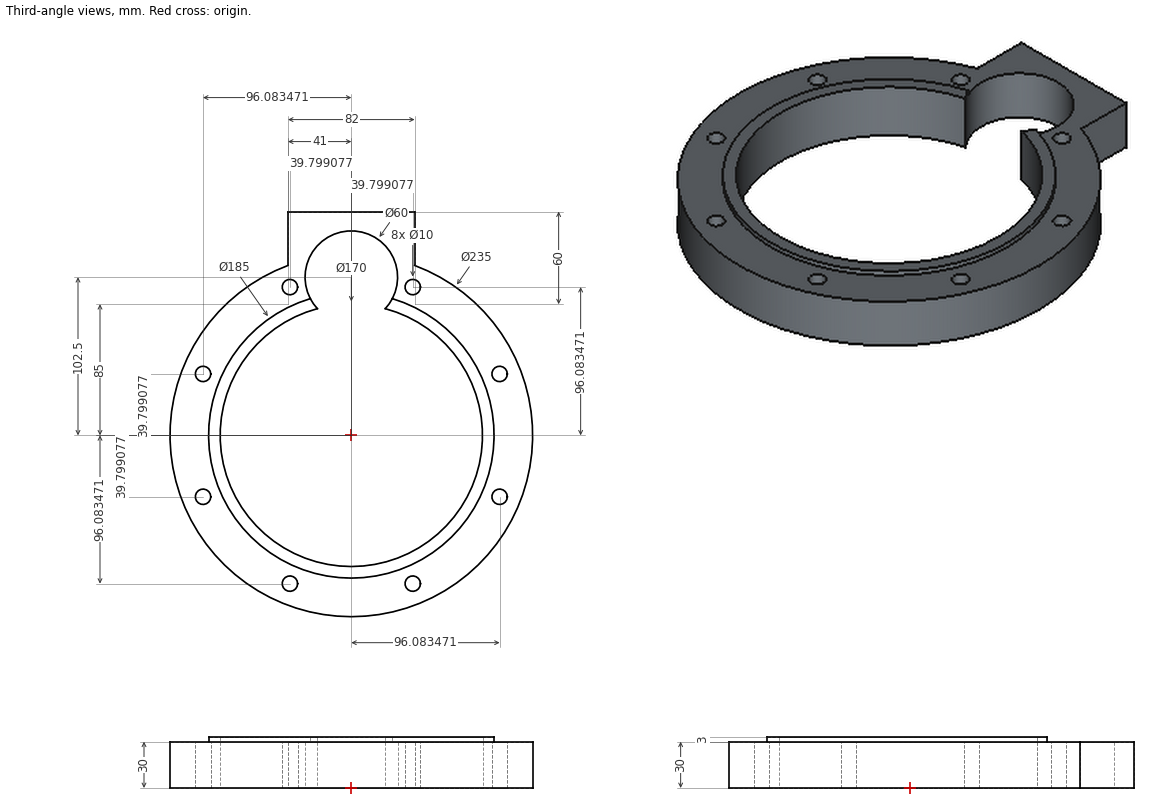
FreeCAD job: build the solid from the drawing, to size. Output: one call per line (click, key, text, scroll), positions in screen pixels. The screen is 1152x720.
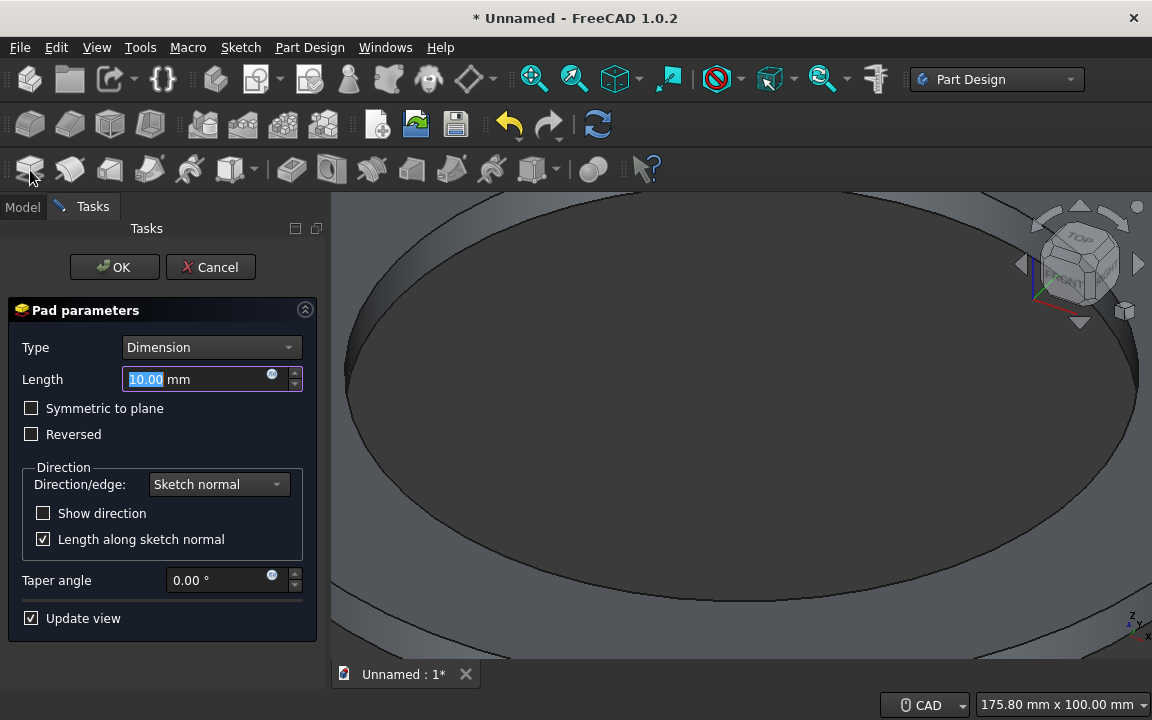
text(30)
key(Tab)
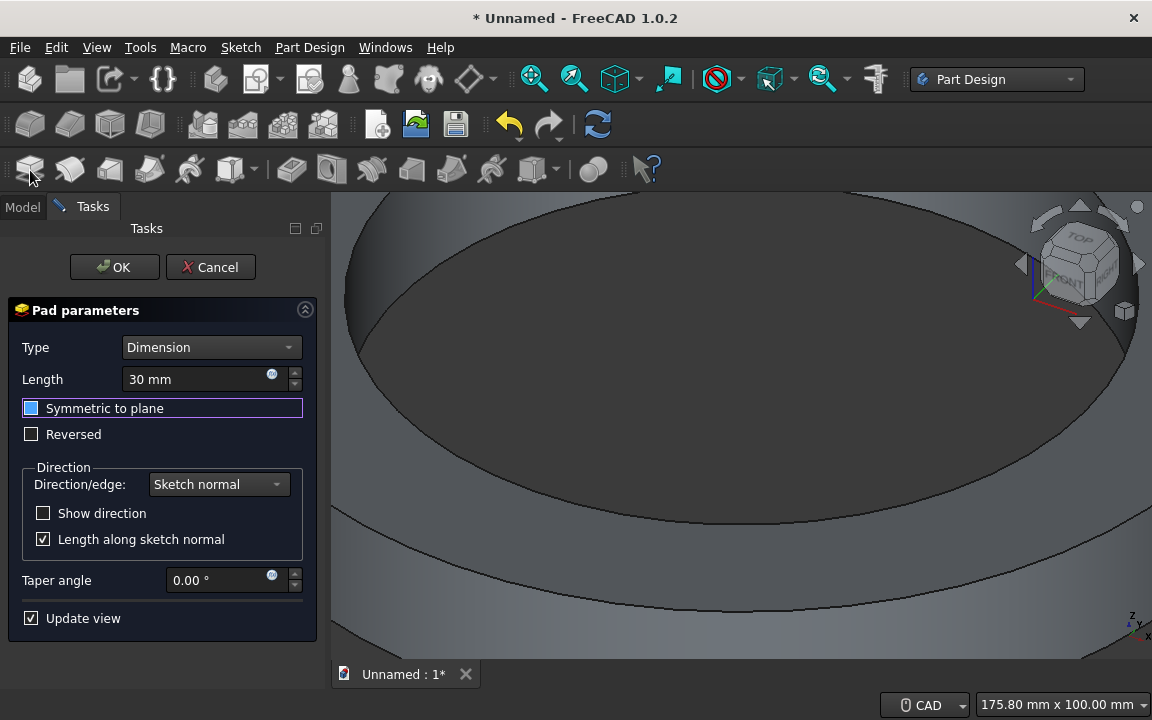
click(115, 267)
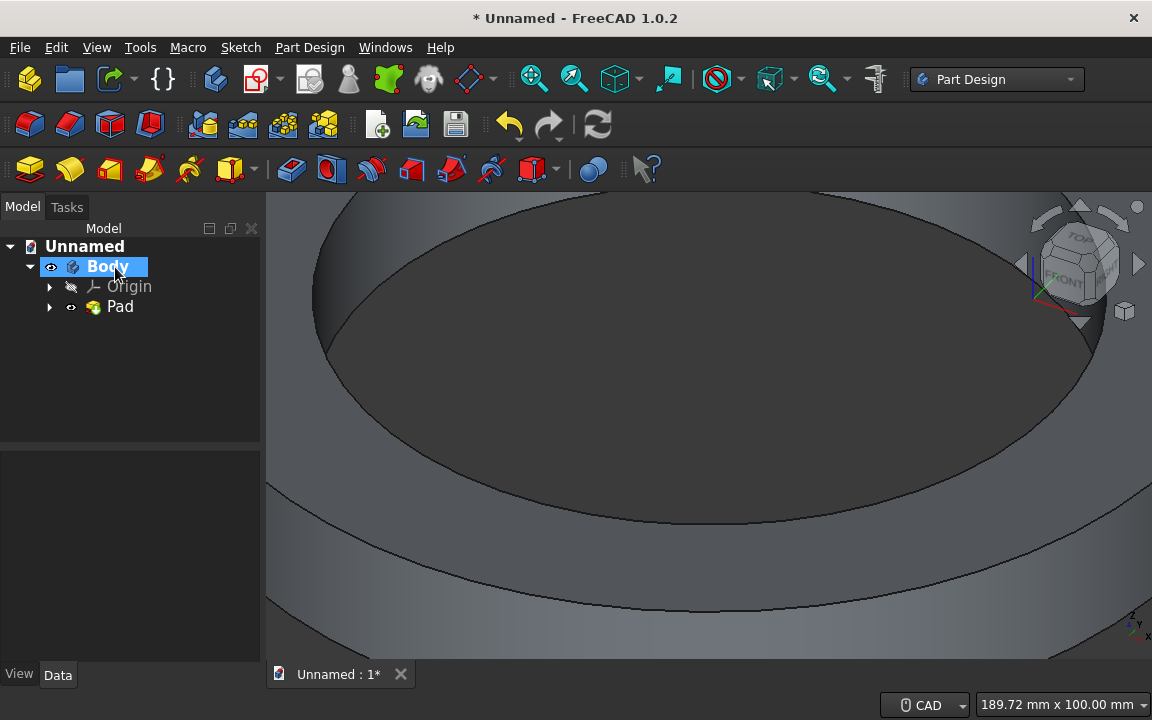
click(536, 80)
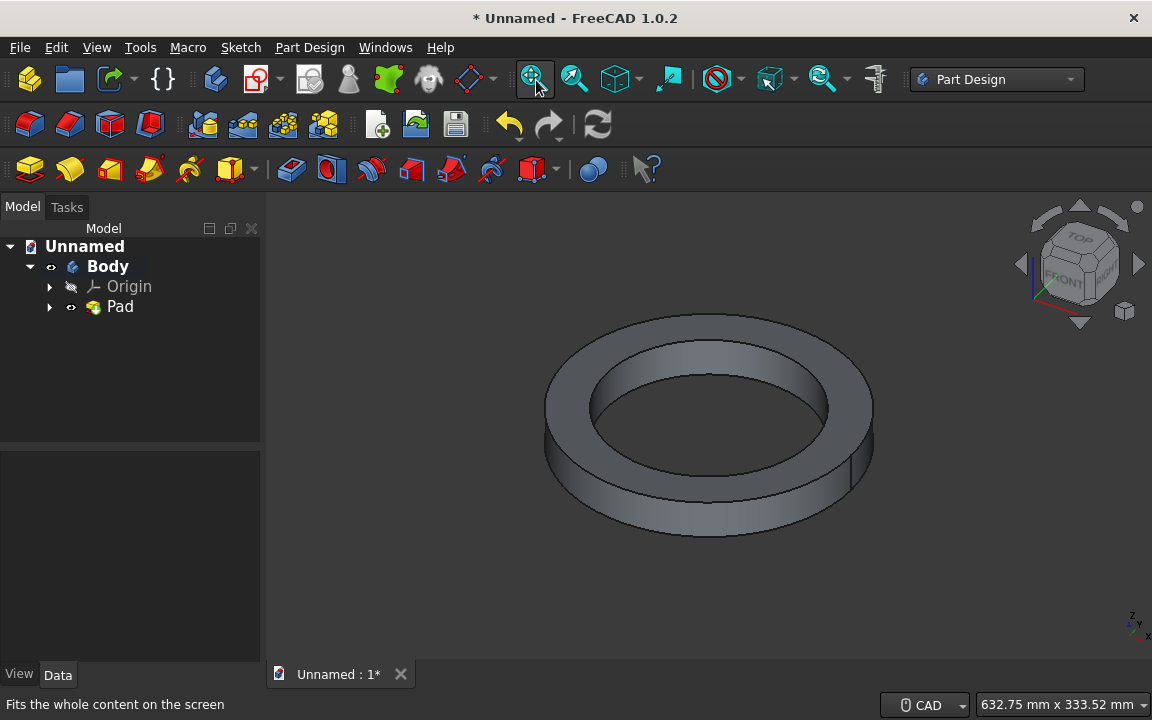
click(831, 448)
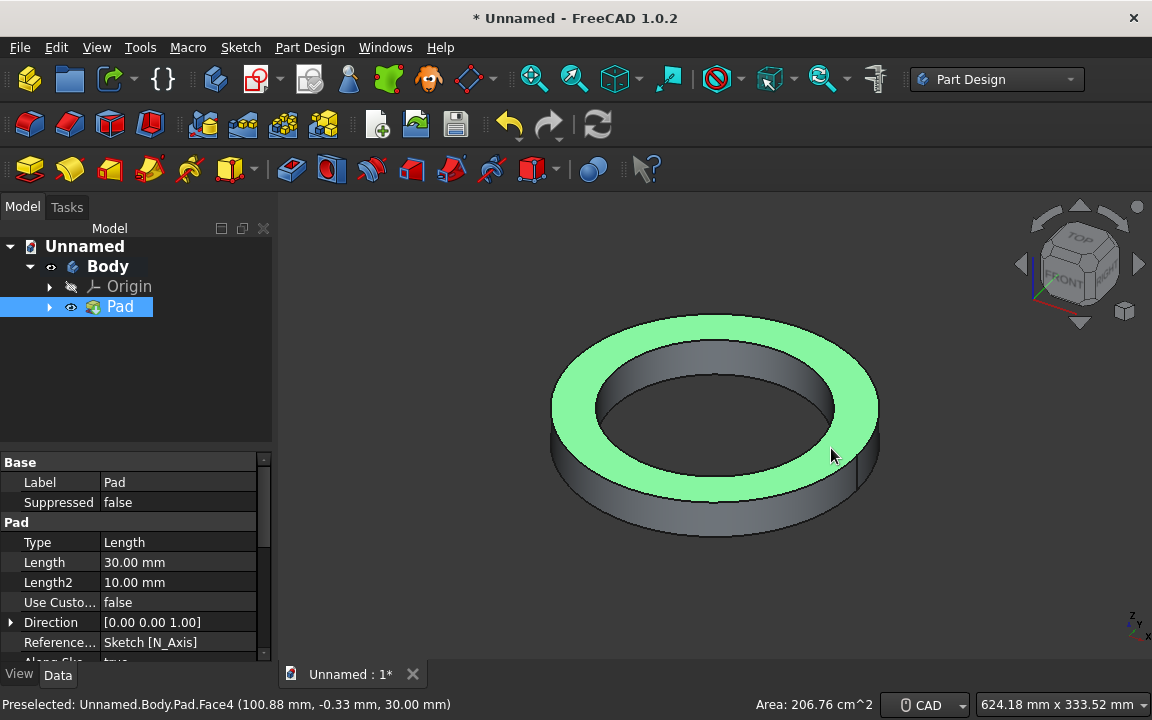
click(256, 80)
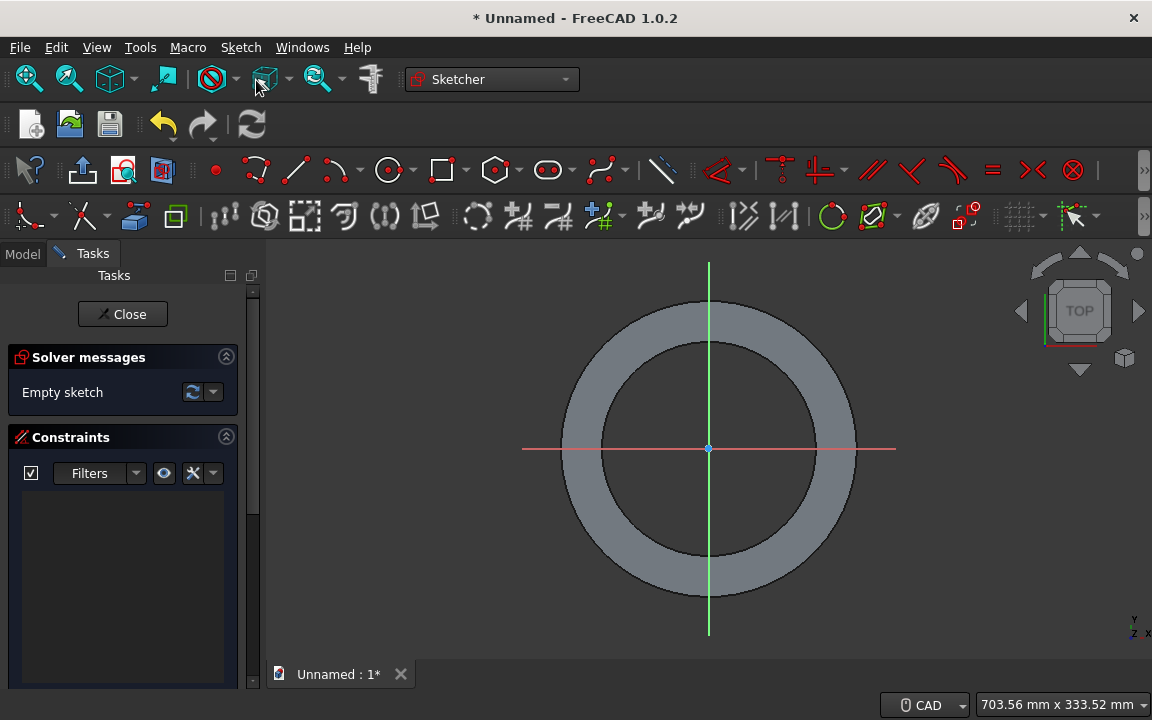
scroll(332, 631, down, 1)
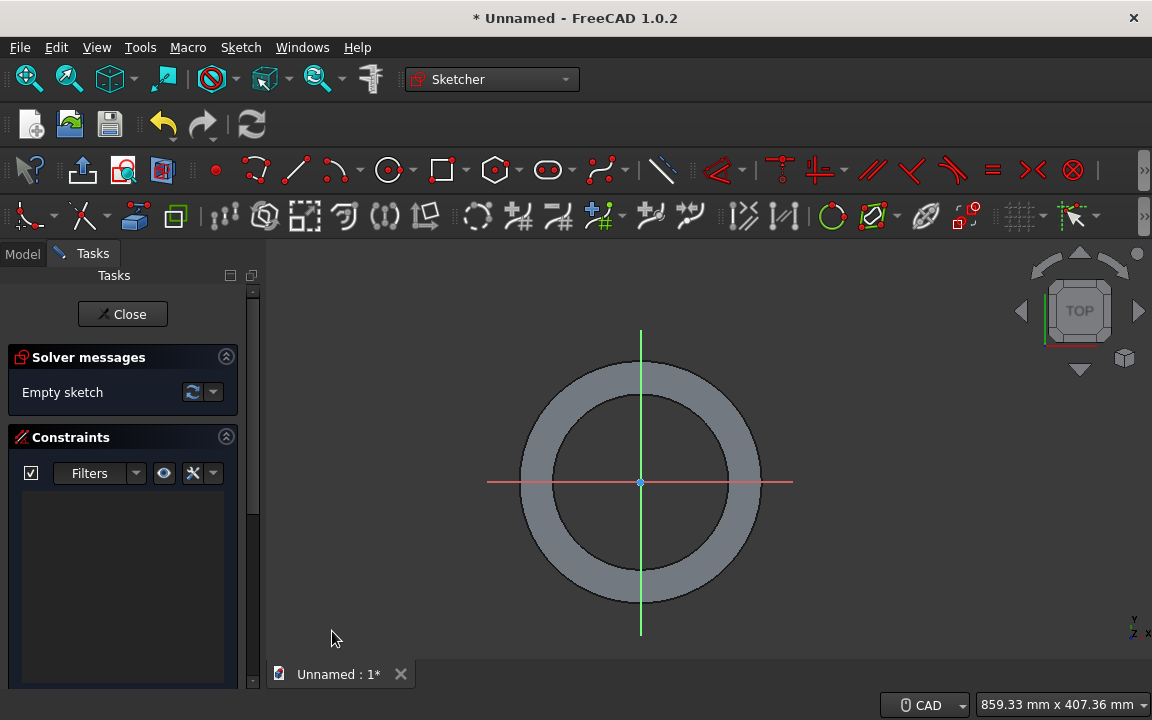
scroll(641, 357, up, 3)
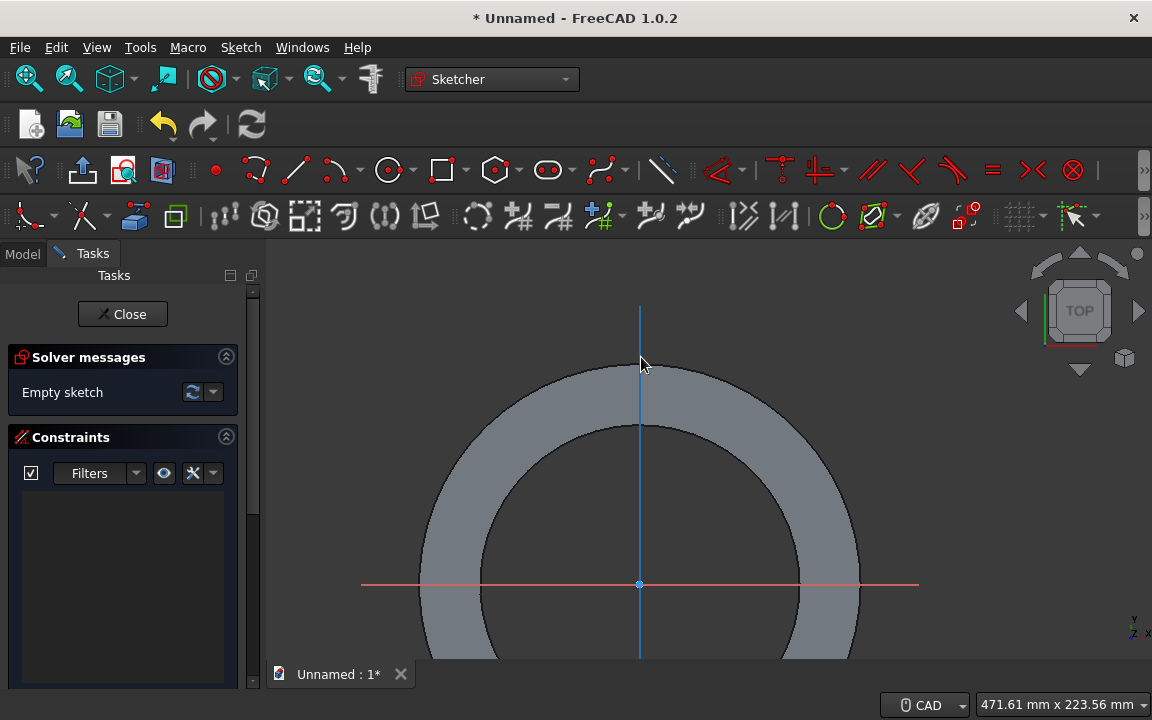
click(442, 170)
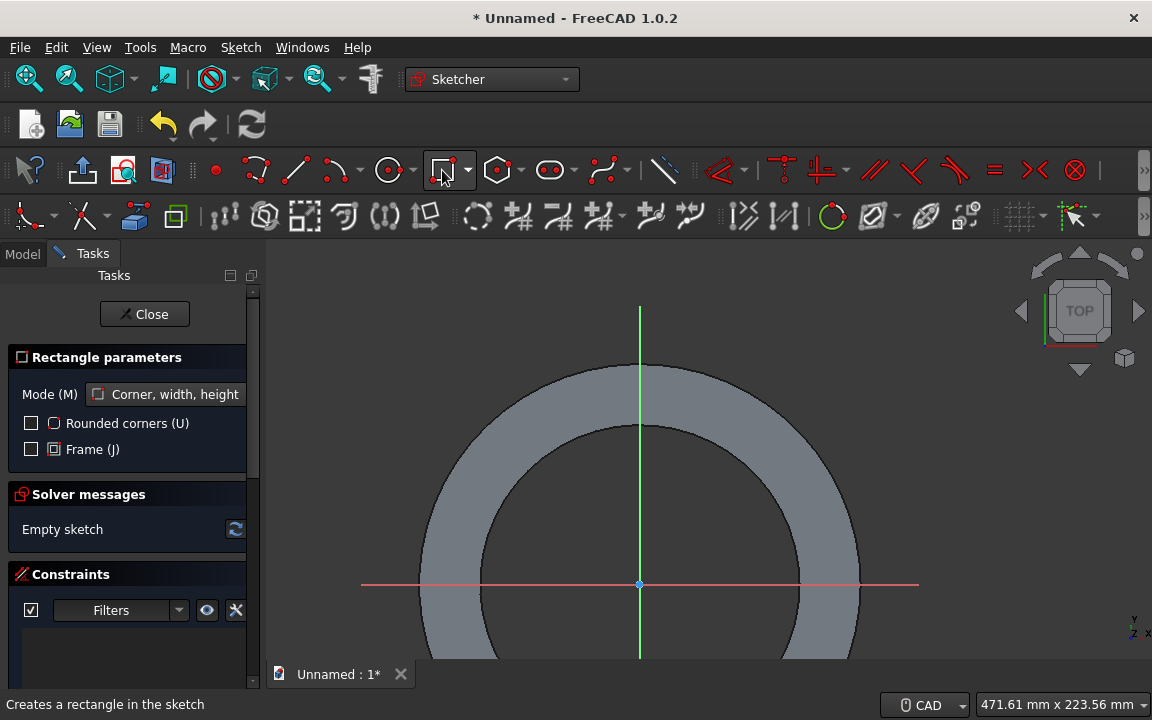
click(563, 312)
move(717, 425)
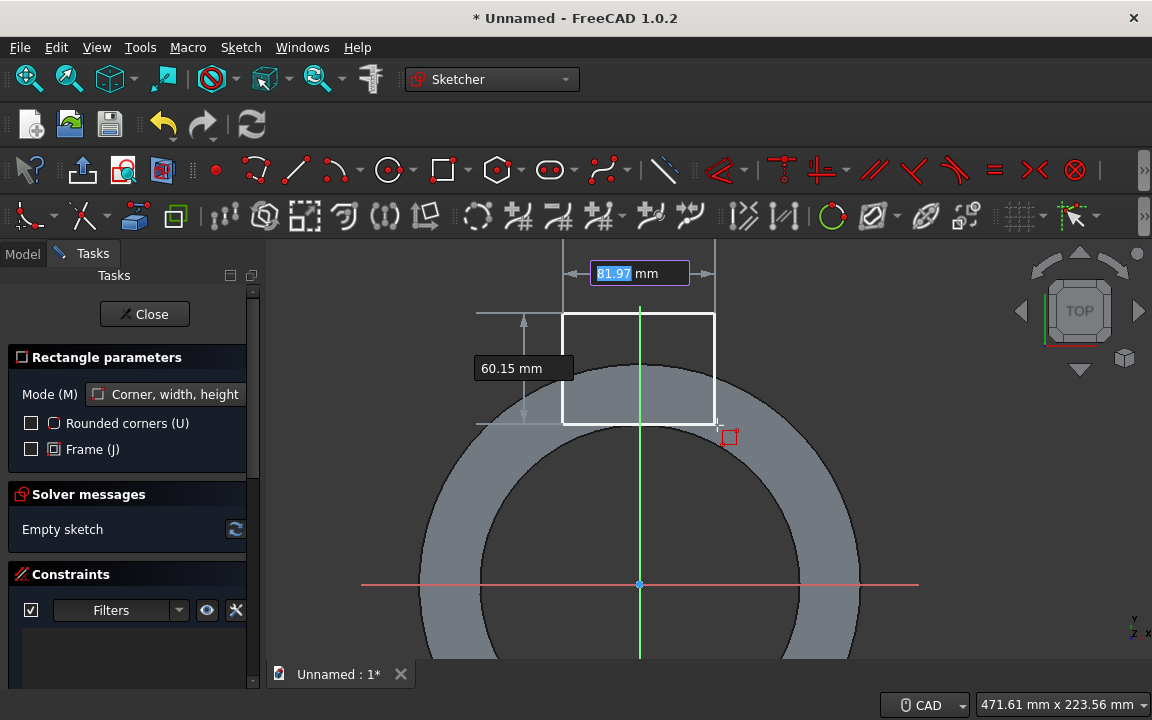
text(82)
key(Tab)
text(60)
key(Return)
key(Escape)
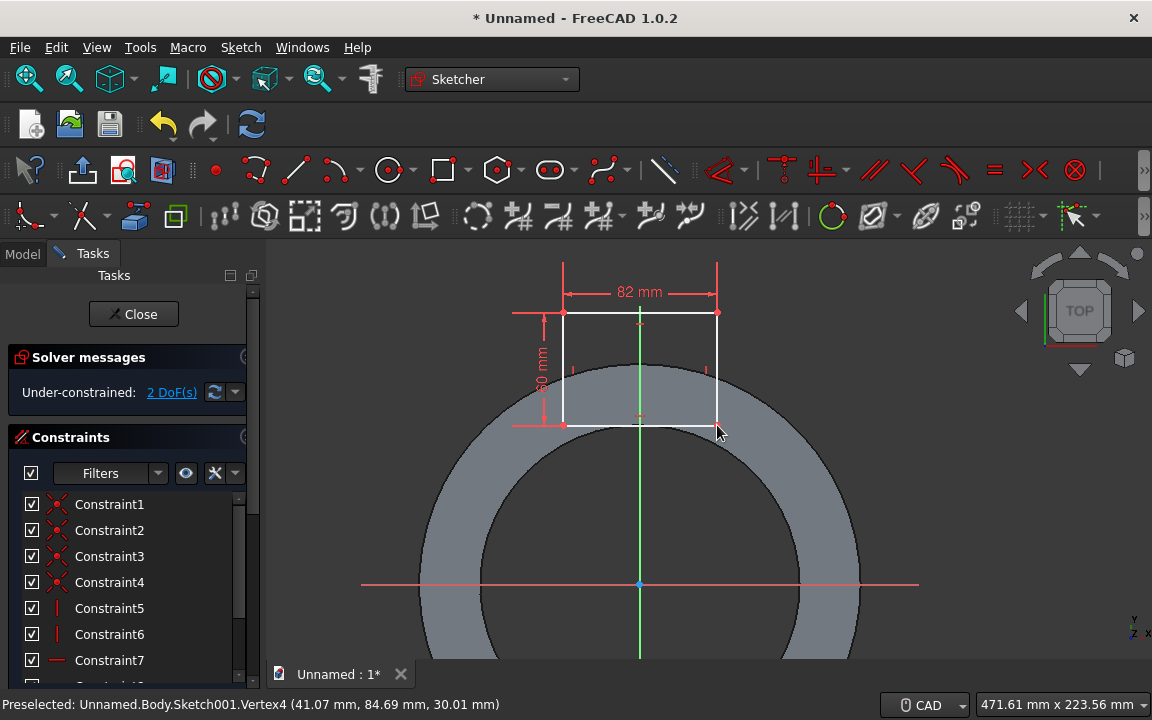
click(563, 313)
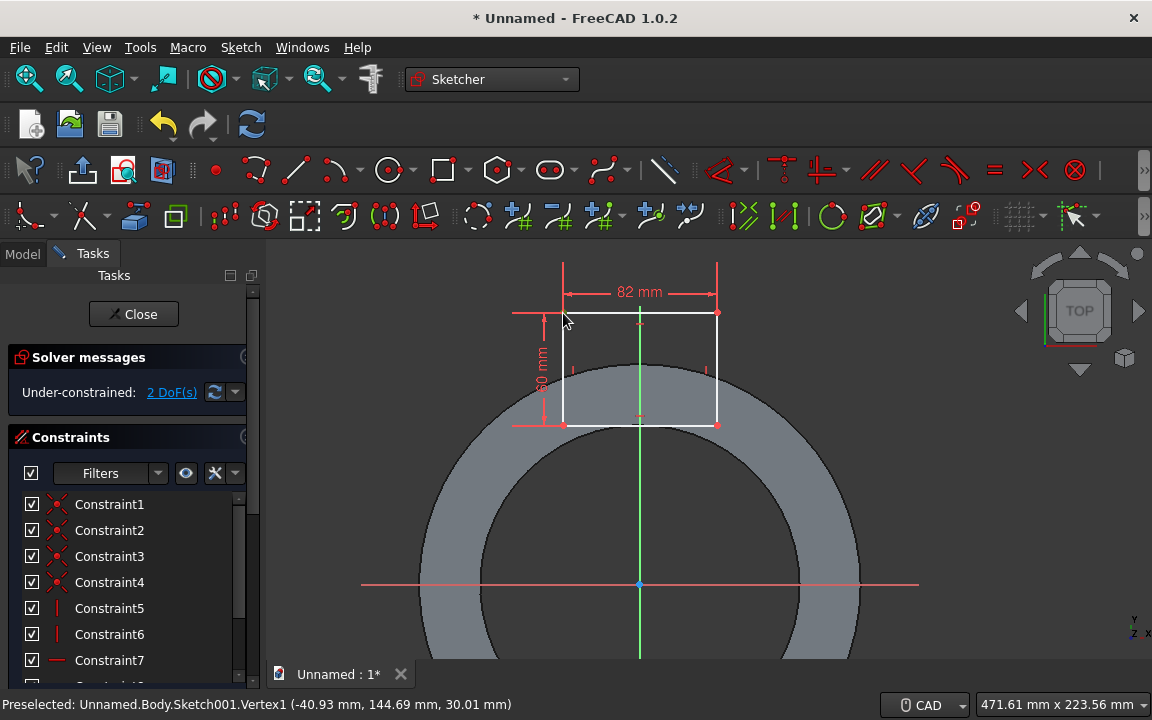
key(l)